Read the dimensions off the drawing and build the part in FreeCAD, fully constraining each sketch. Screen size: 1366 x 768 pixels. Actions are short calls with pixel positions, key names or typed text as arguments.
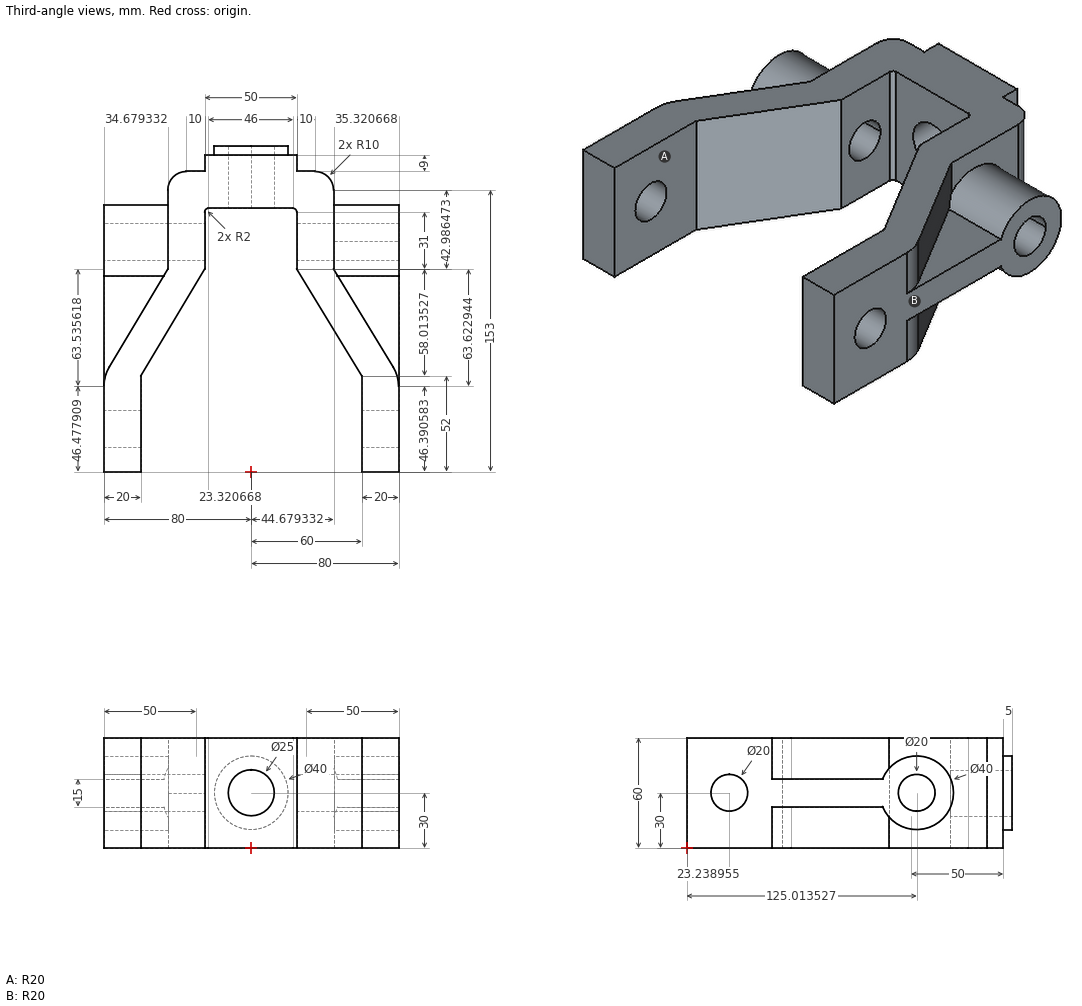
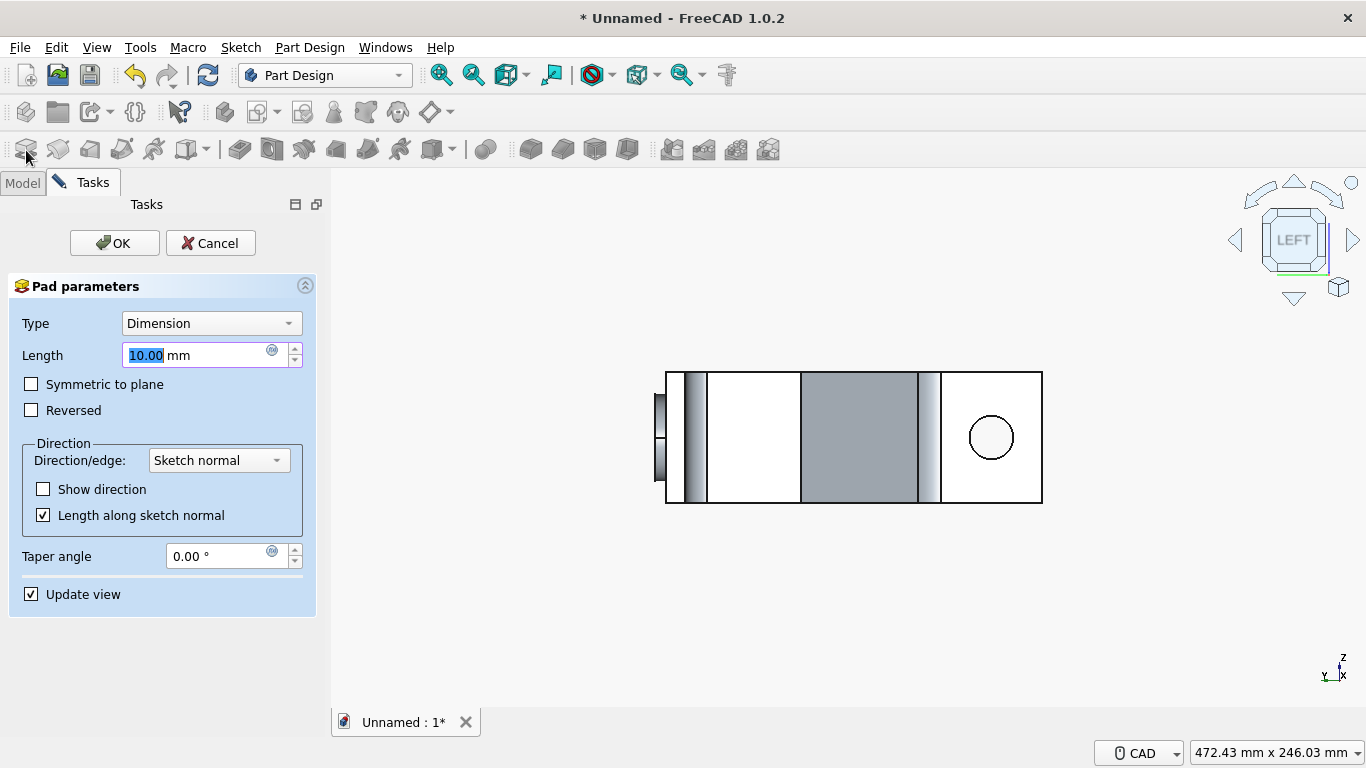
text(50)
key(Tab)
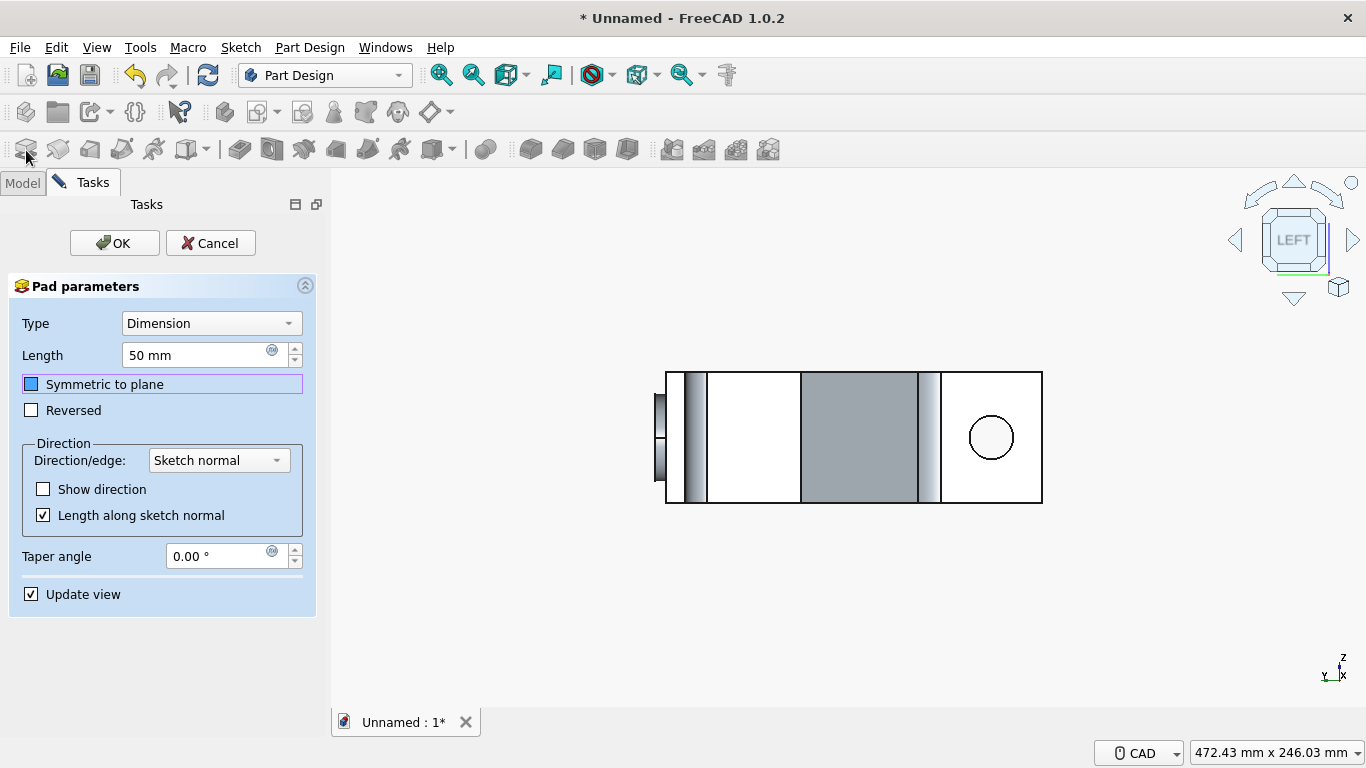
click(30, 410)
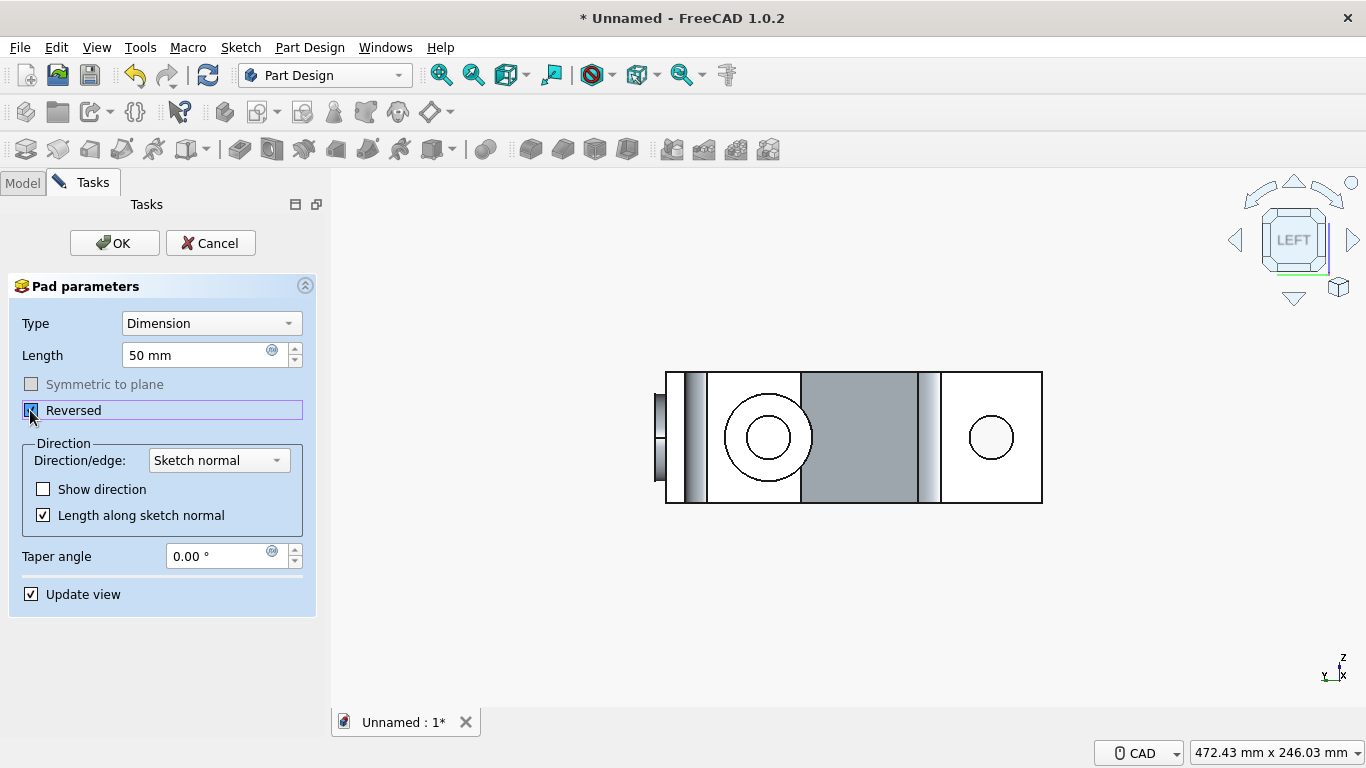
click(115, 243)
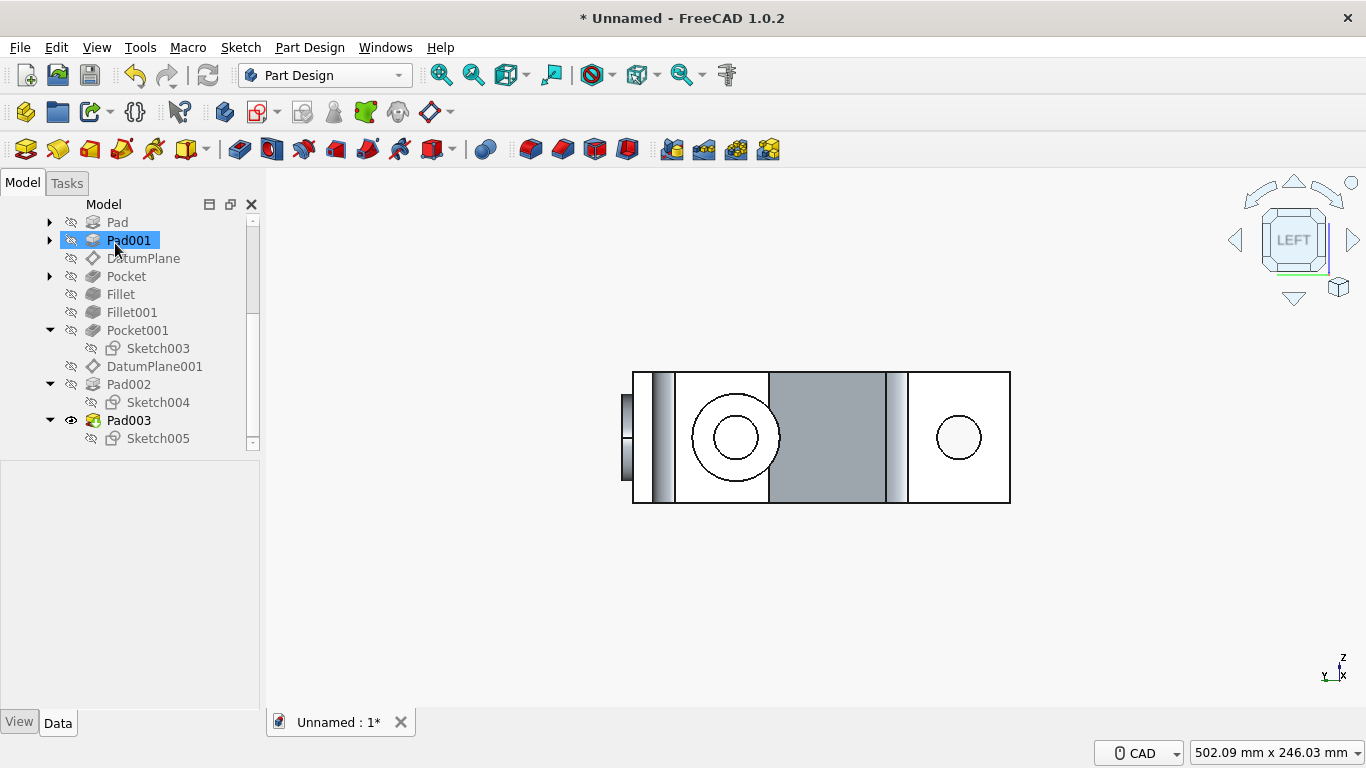
click(442, 76)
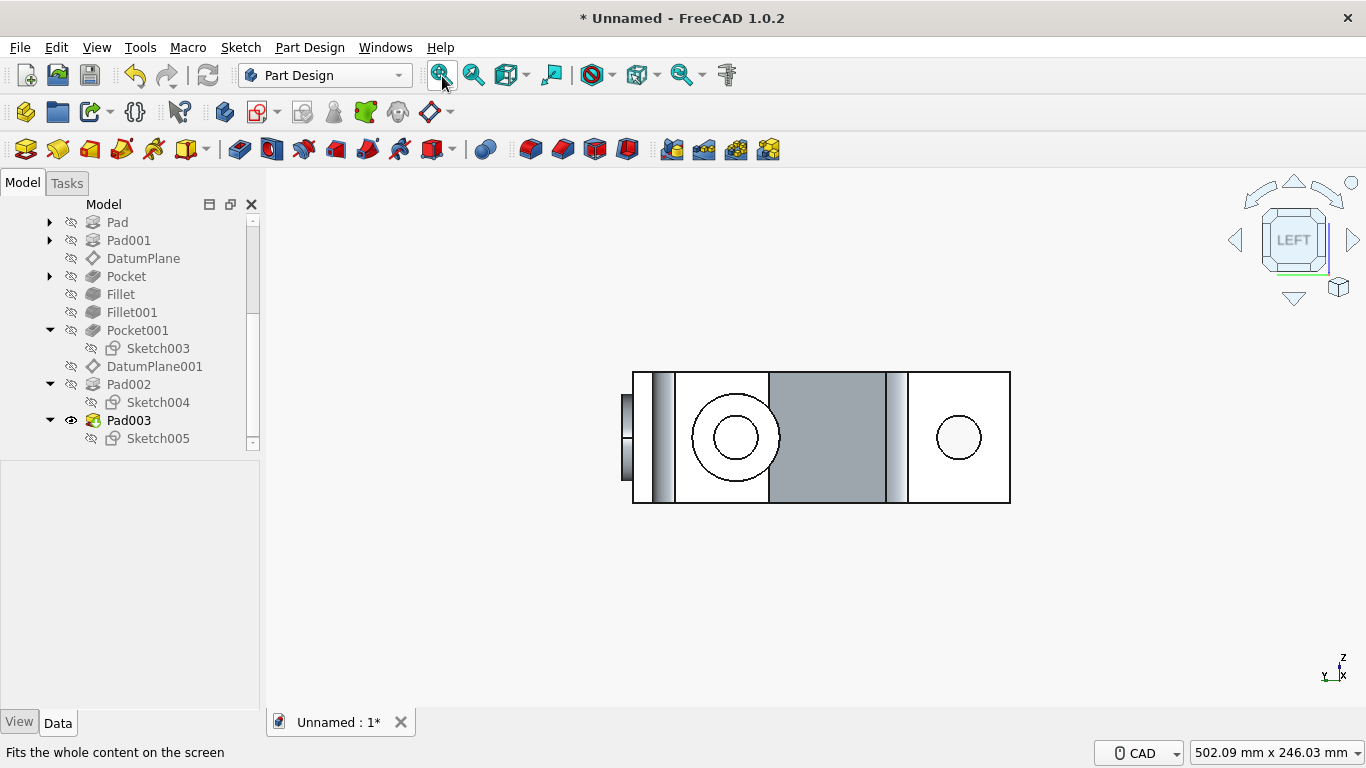
scroll(140, 326, down, 3)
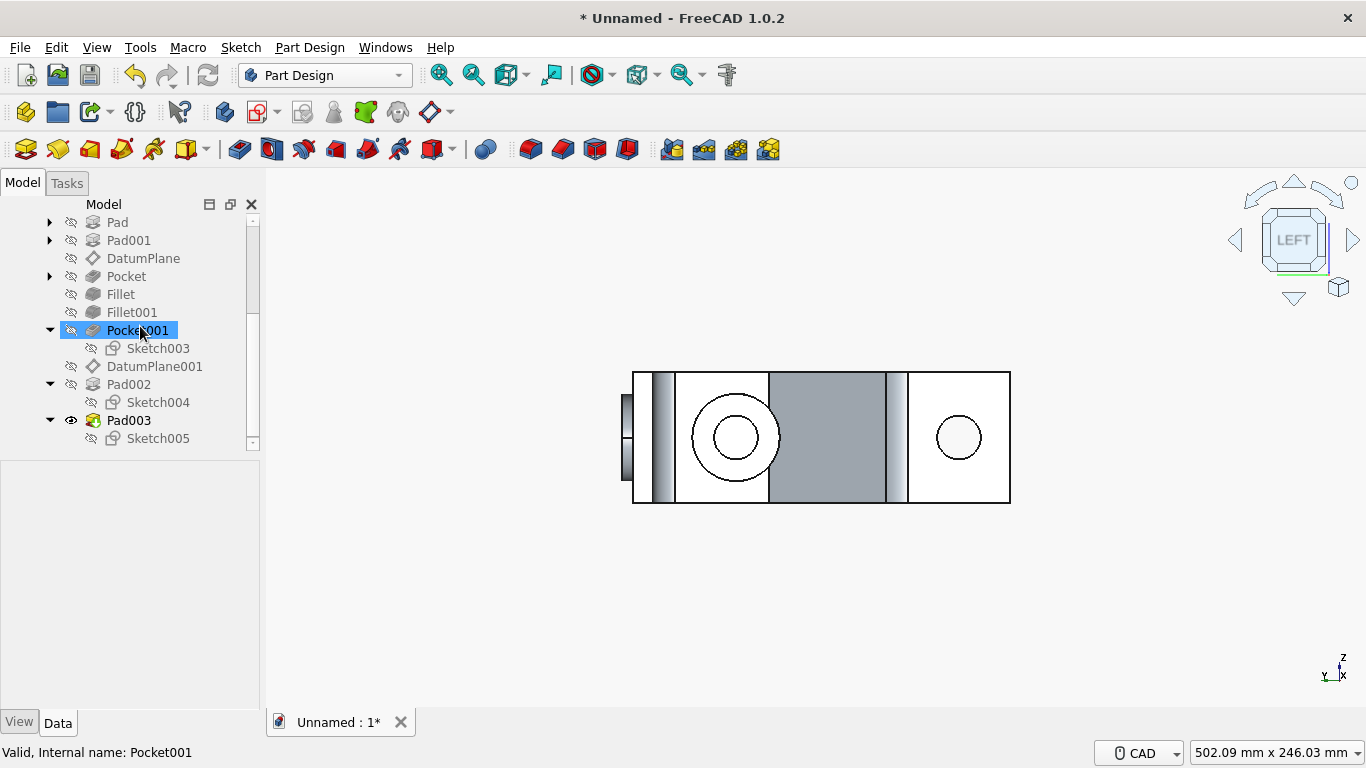
scroll(140, 326, up, 15)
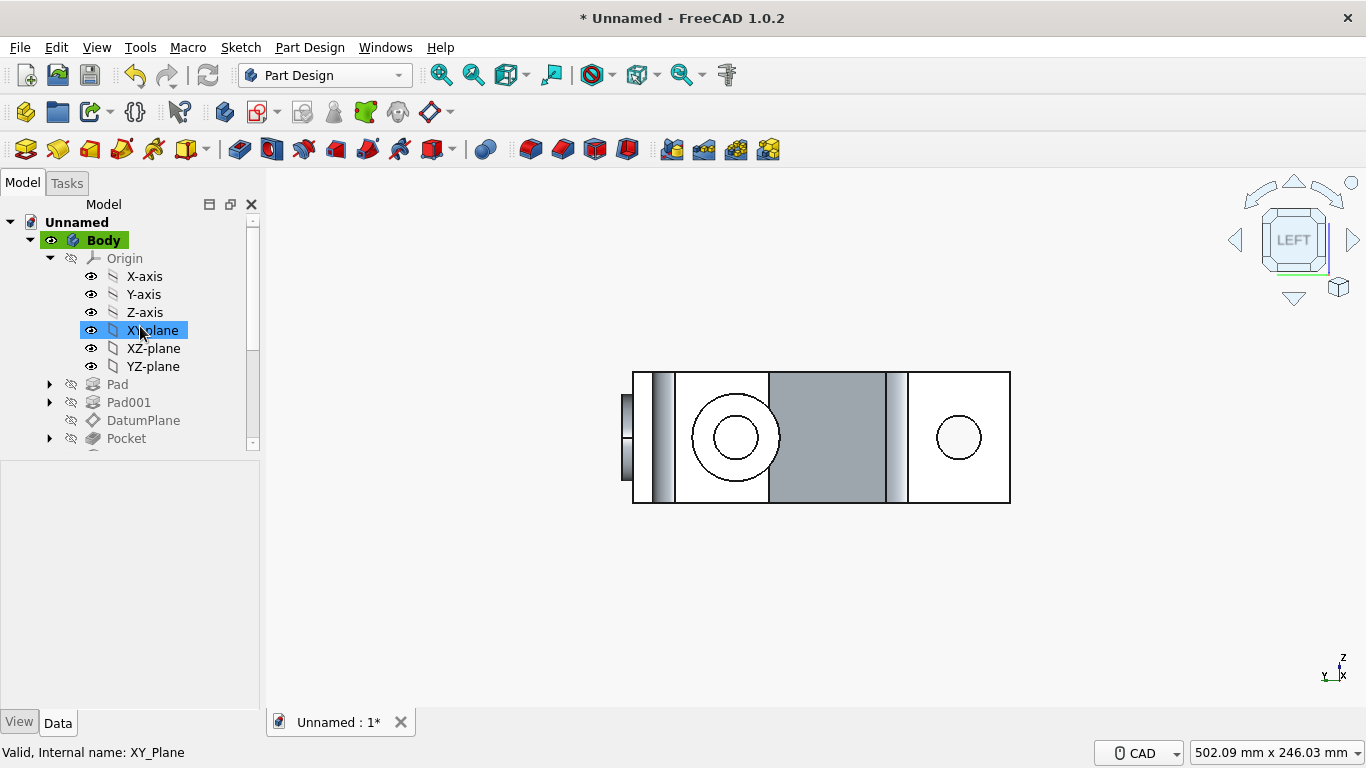
click(136, 366)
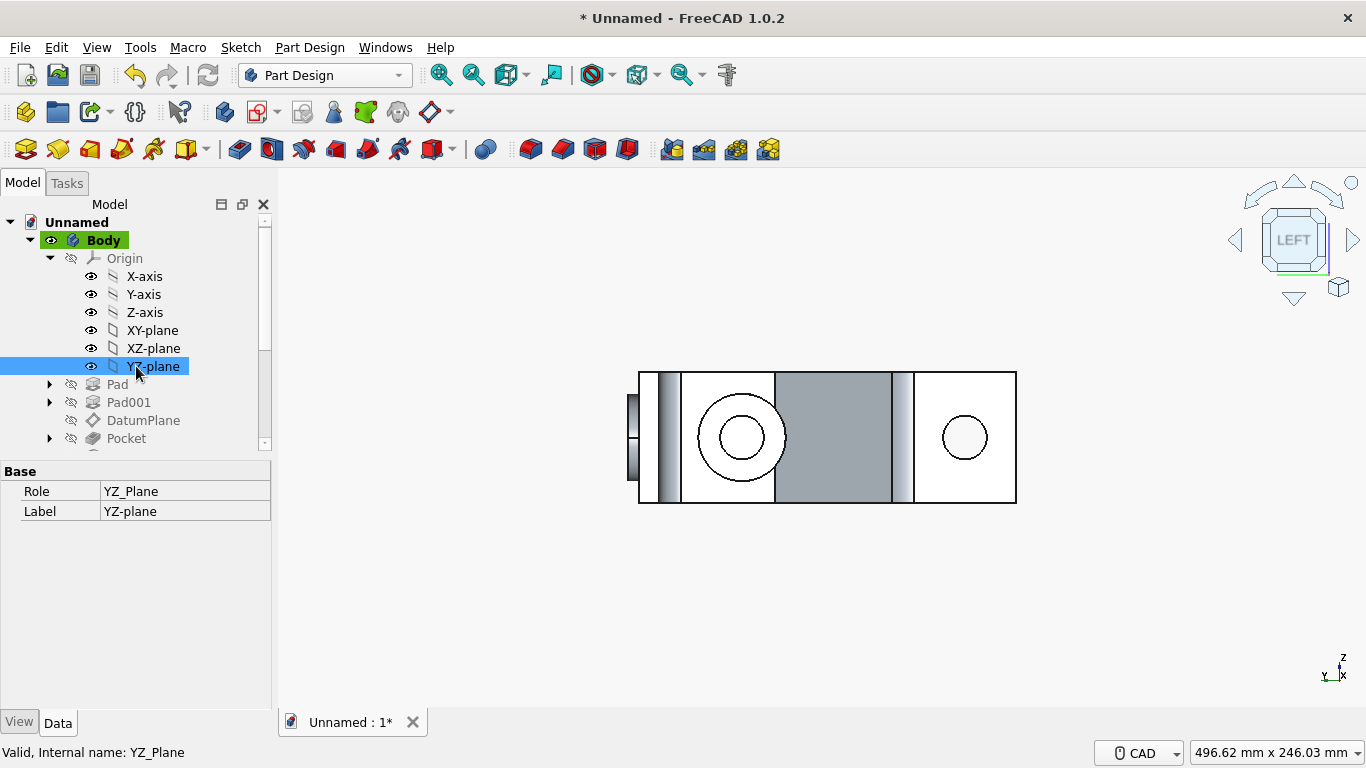
click(430, 112)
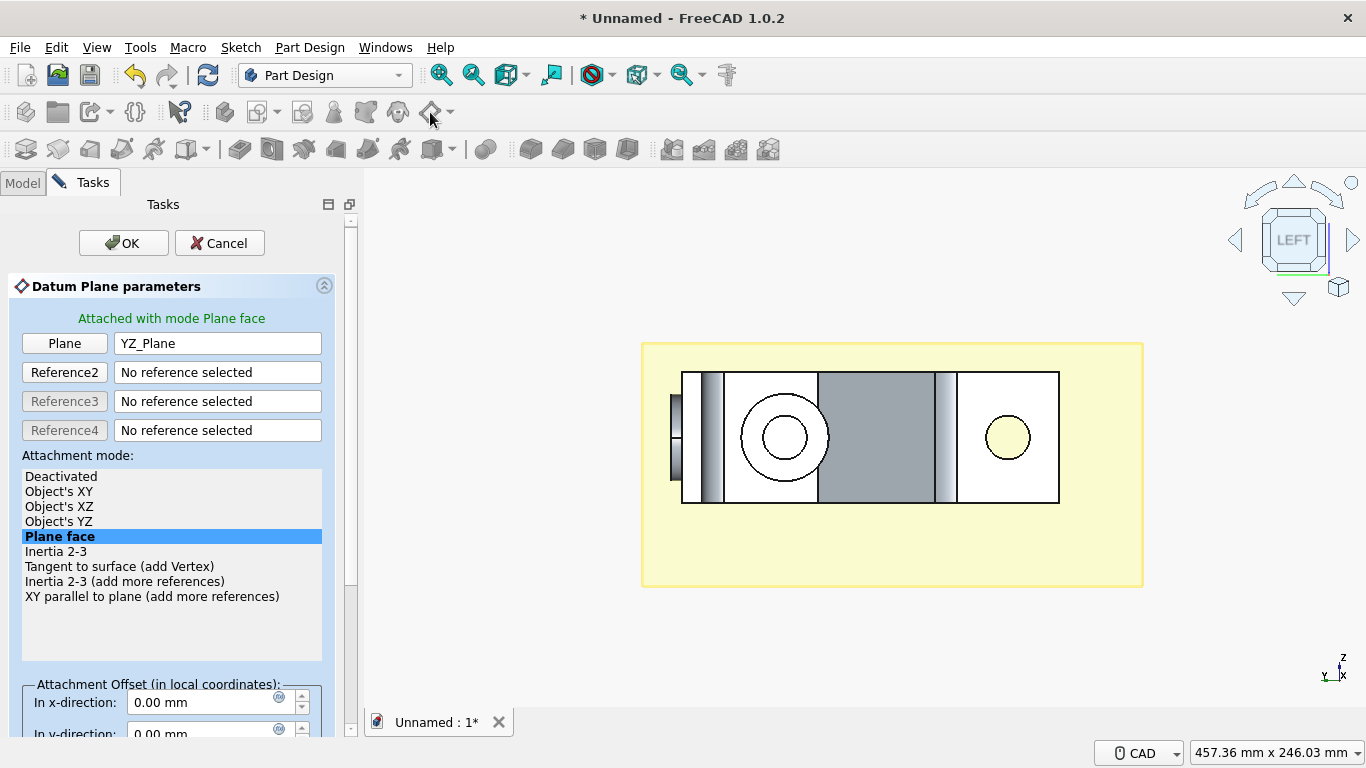
scroll(351, 475, down, 2)